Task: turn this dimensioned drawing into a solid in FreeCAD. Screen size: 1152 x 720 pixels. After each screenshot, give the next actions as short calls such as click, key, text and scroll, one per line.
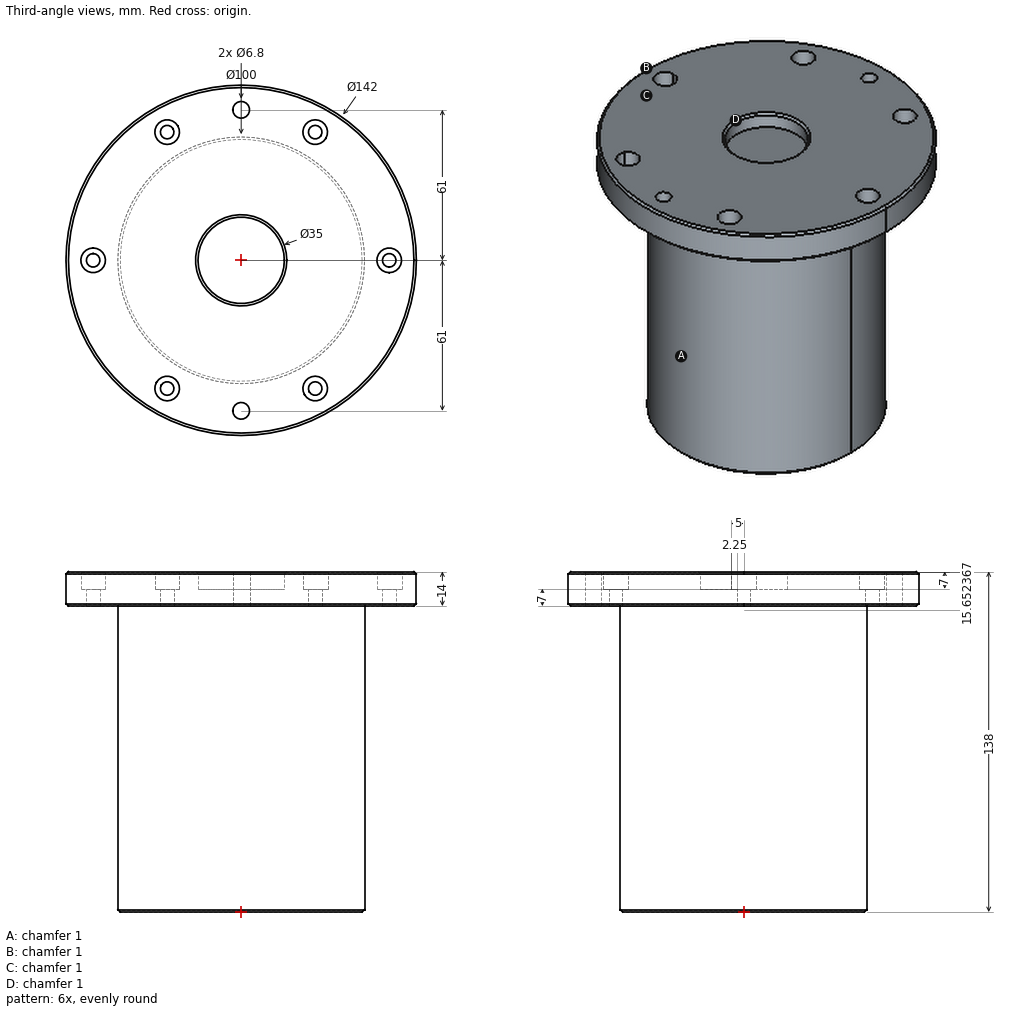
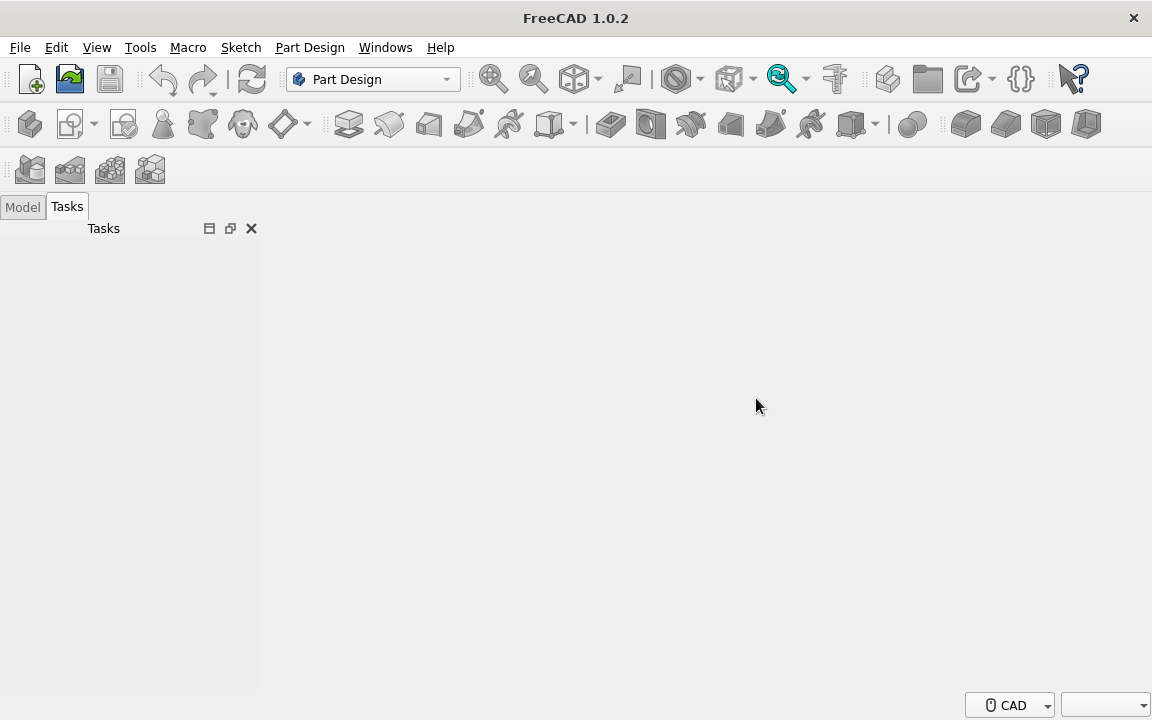
click(30, 80)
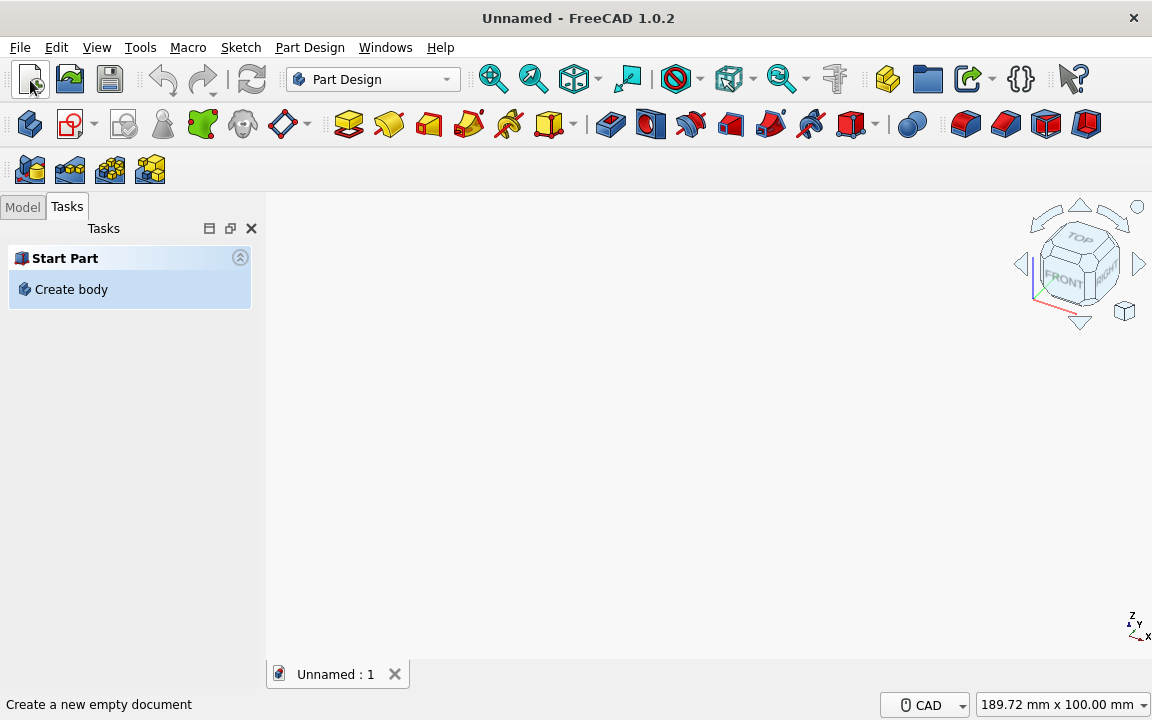
click(70, 124)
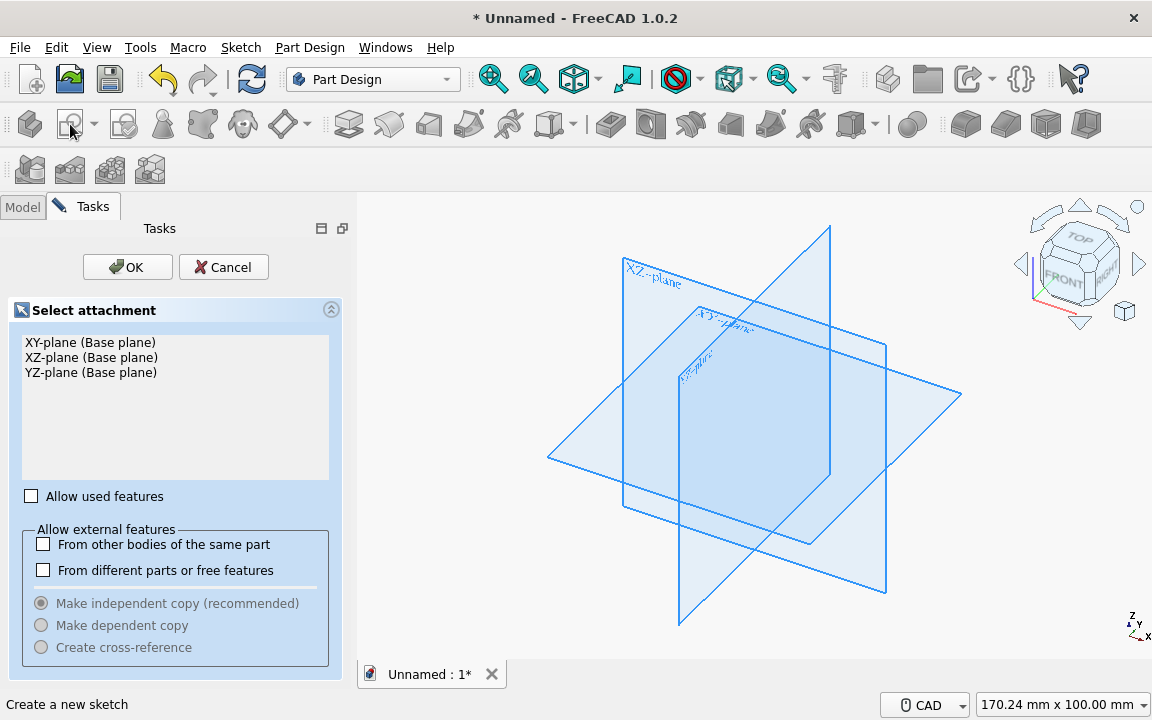
click(82, 342)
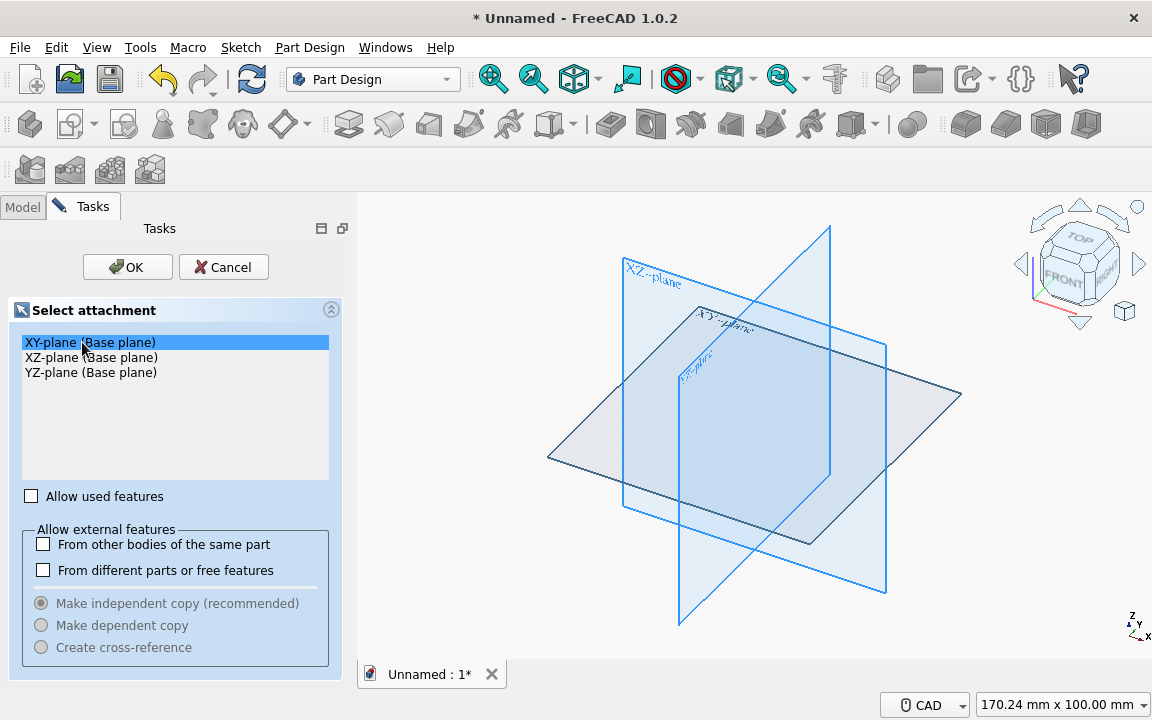
click(128, 267)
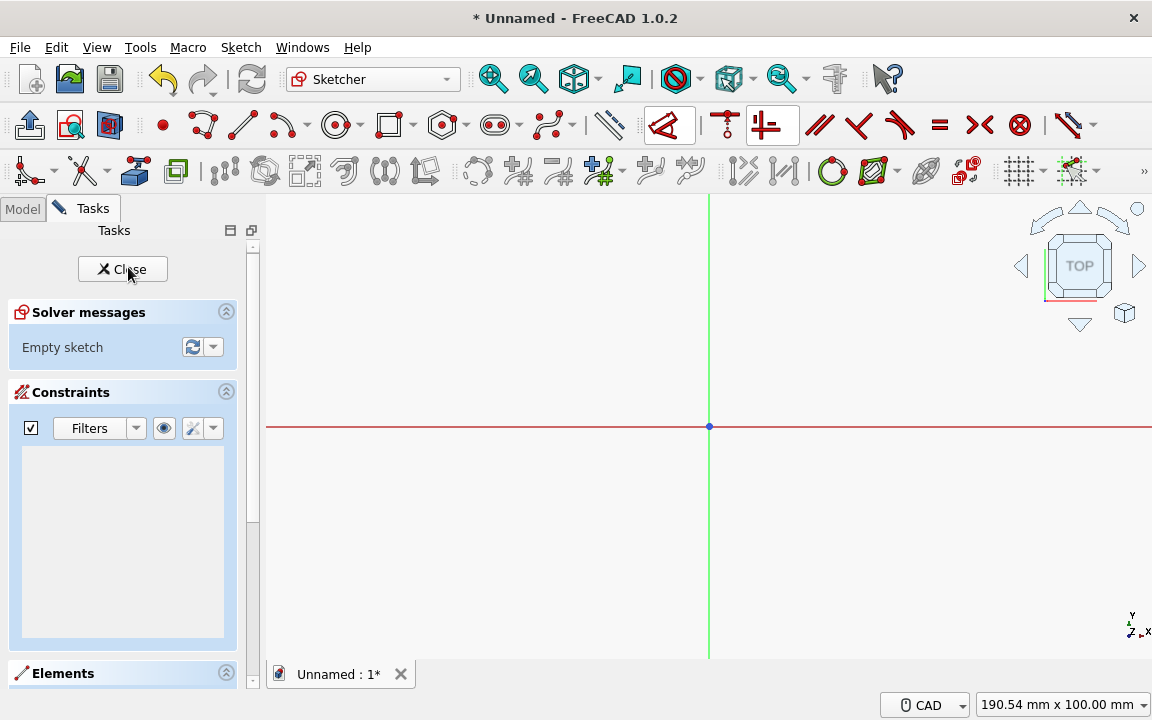
scroll(501, 427, down, 2)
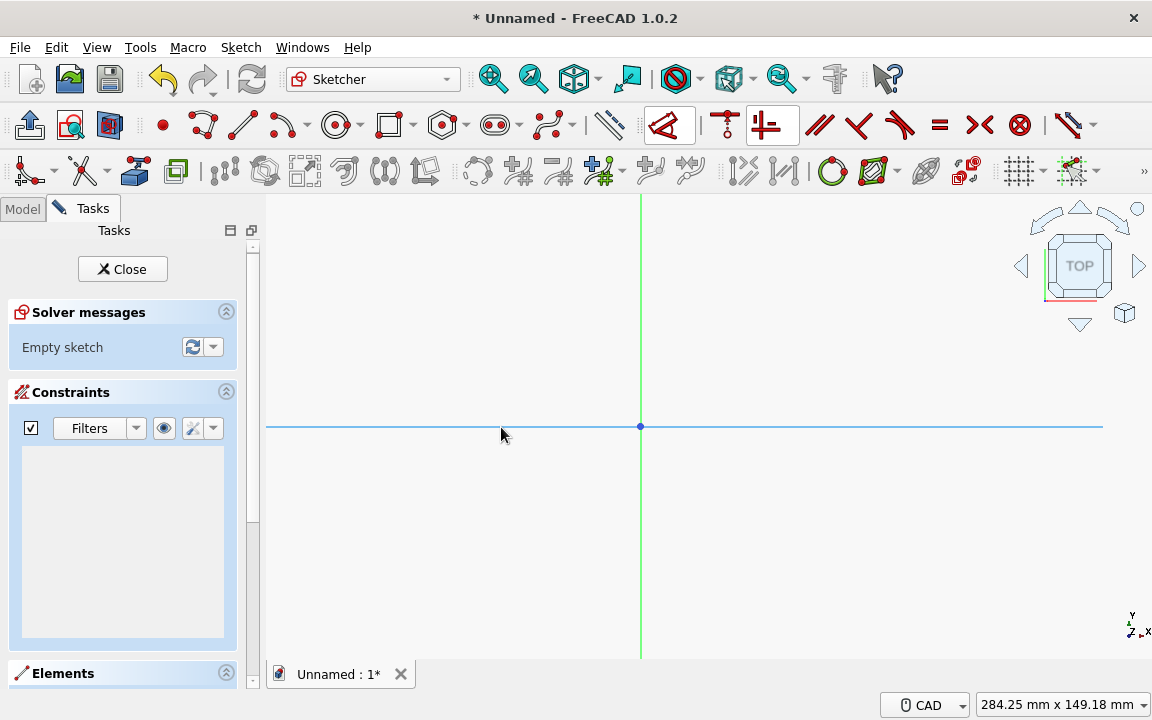
key(g)
key(c)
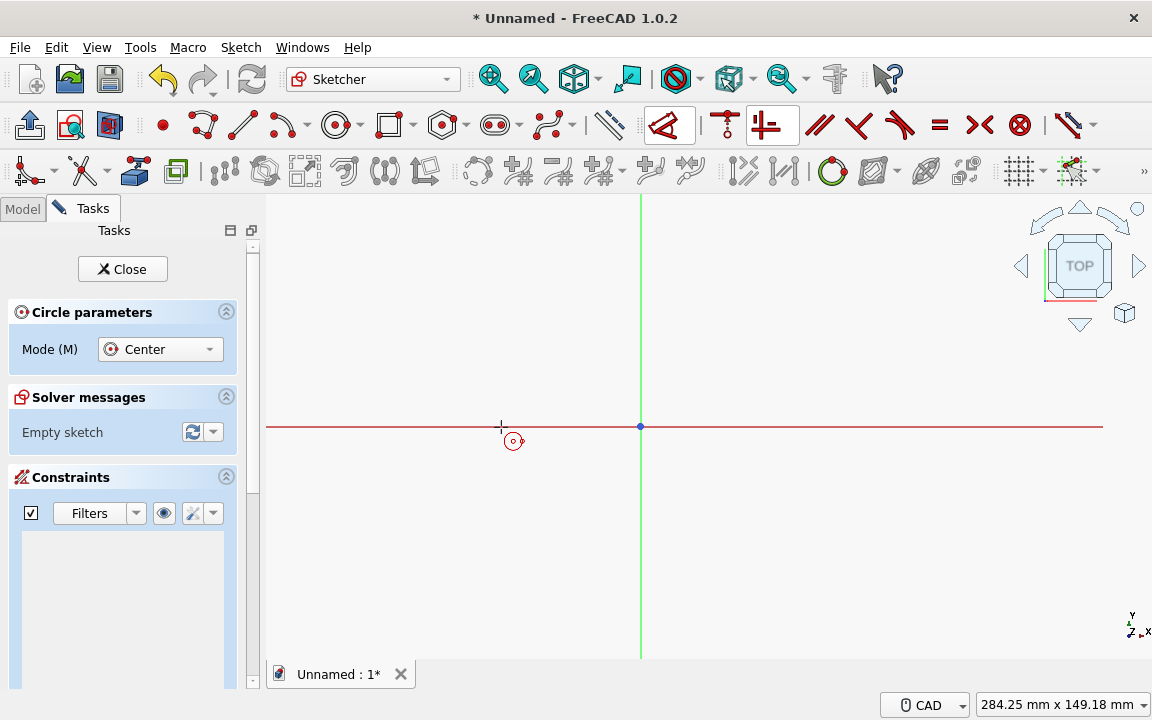
click(641, 427)
click(751, 317)
key(Escape)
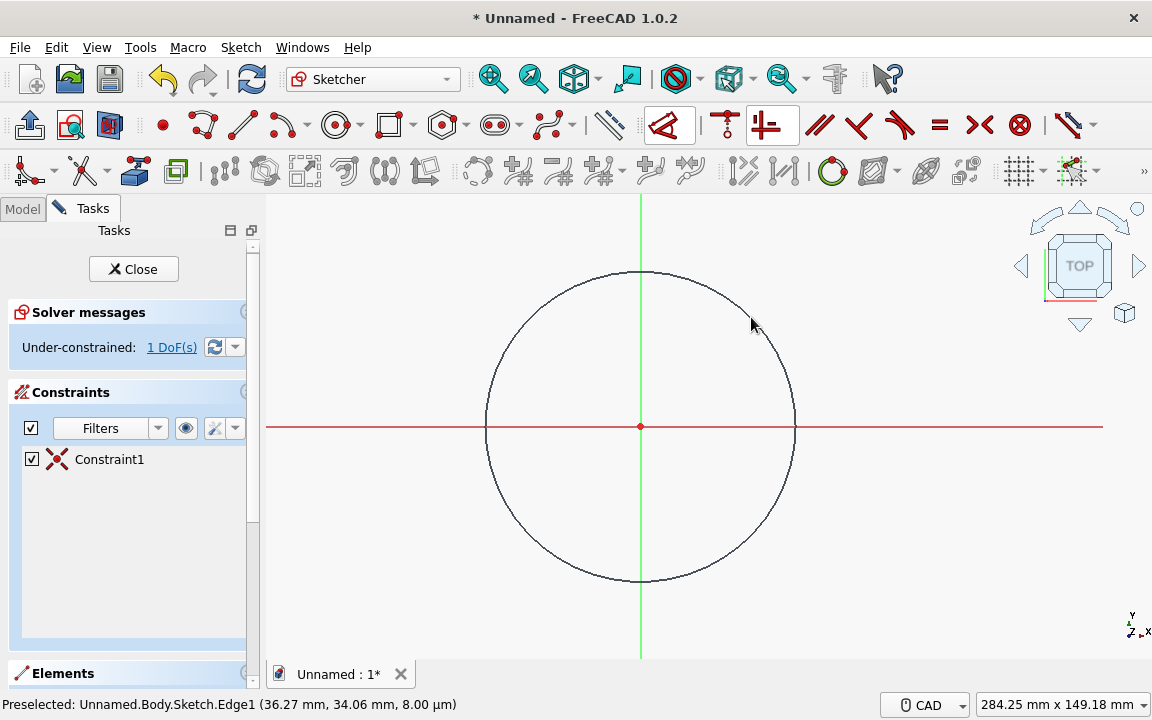
click(750, 317)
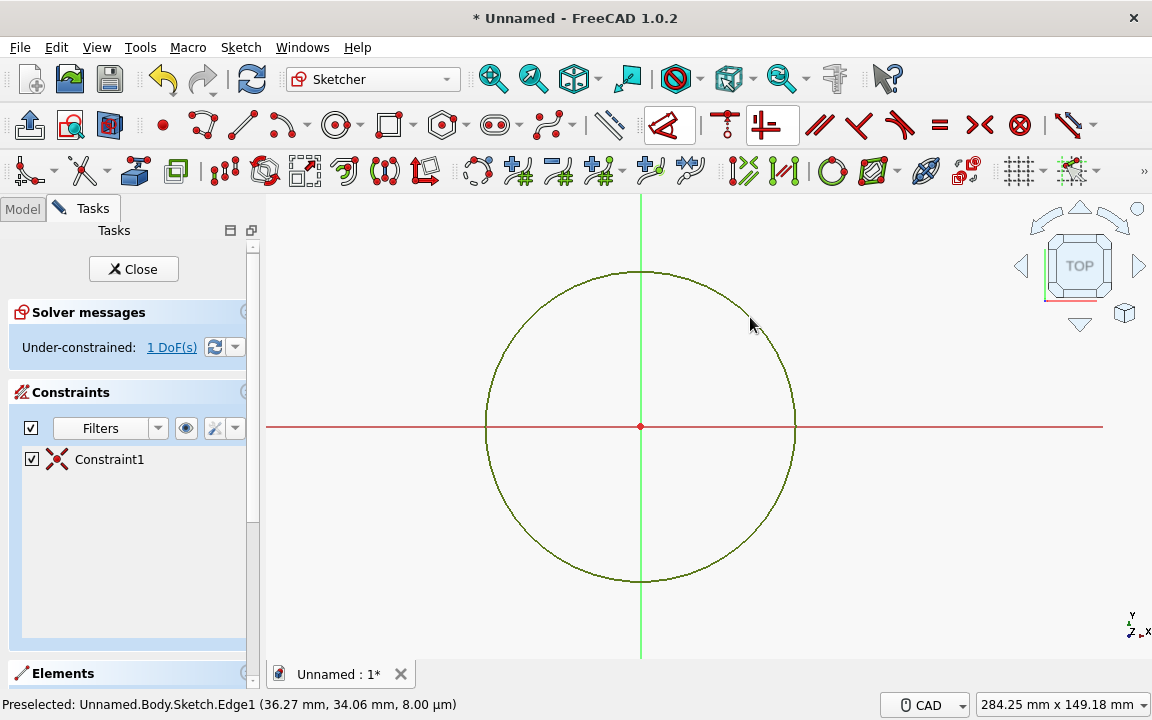
key(k)
key(o)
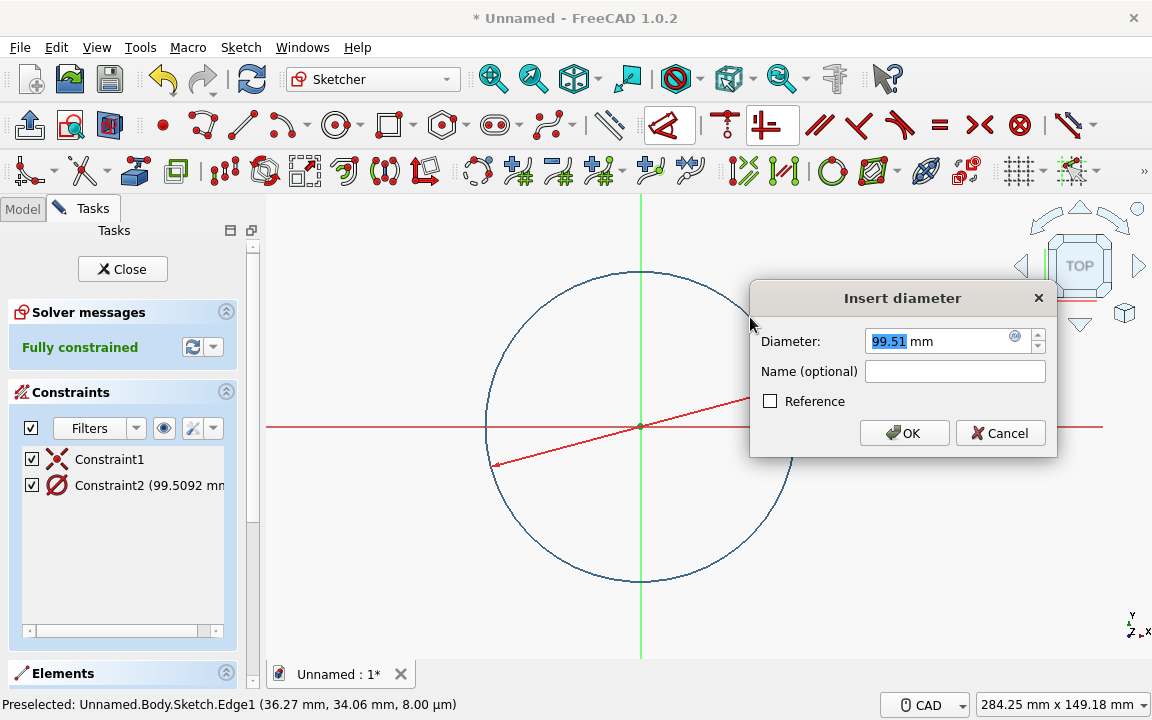
text(100)
key(Return)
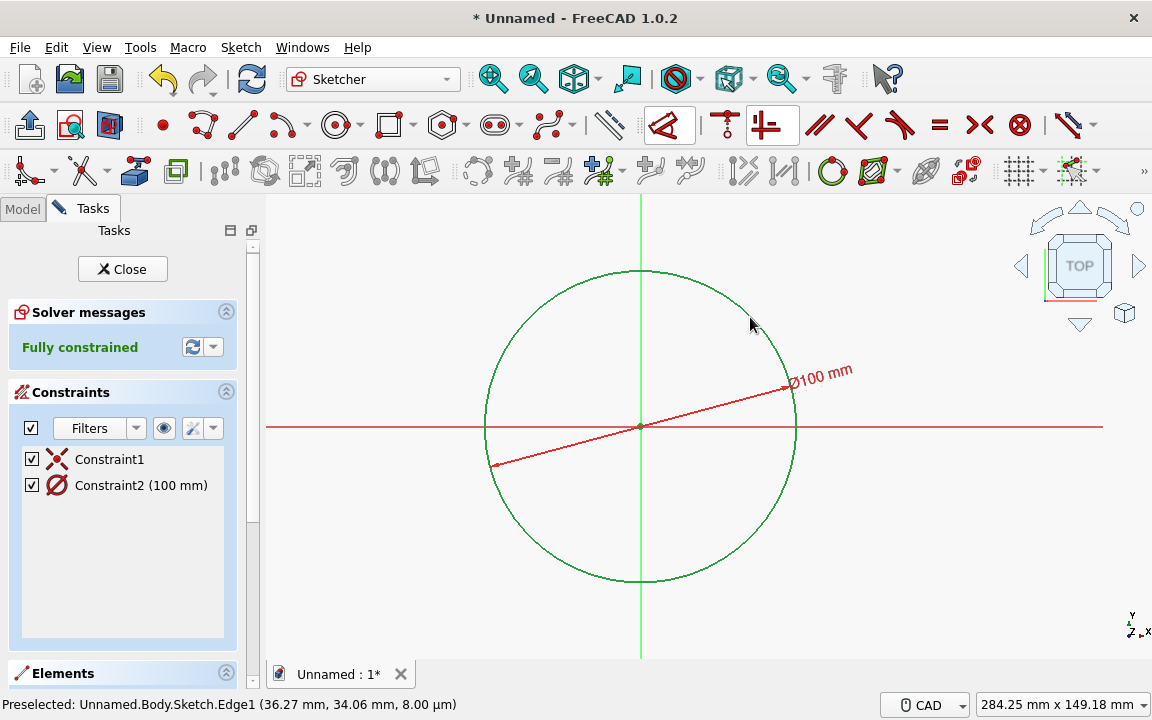
click(123, 269)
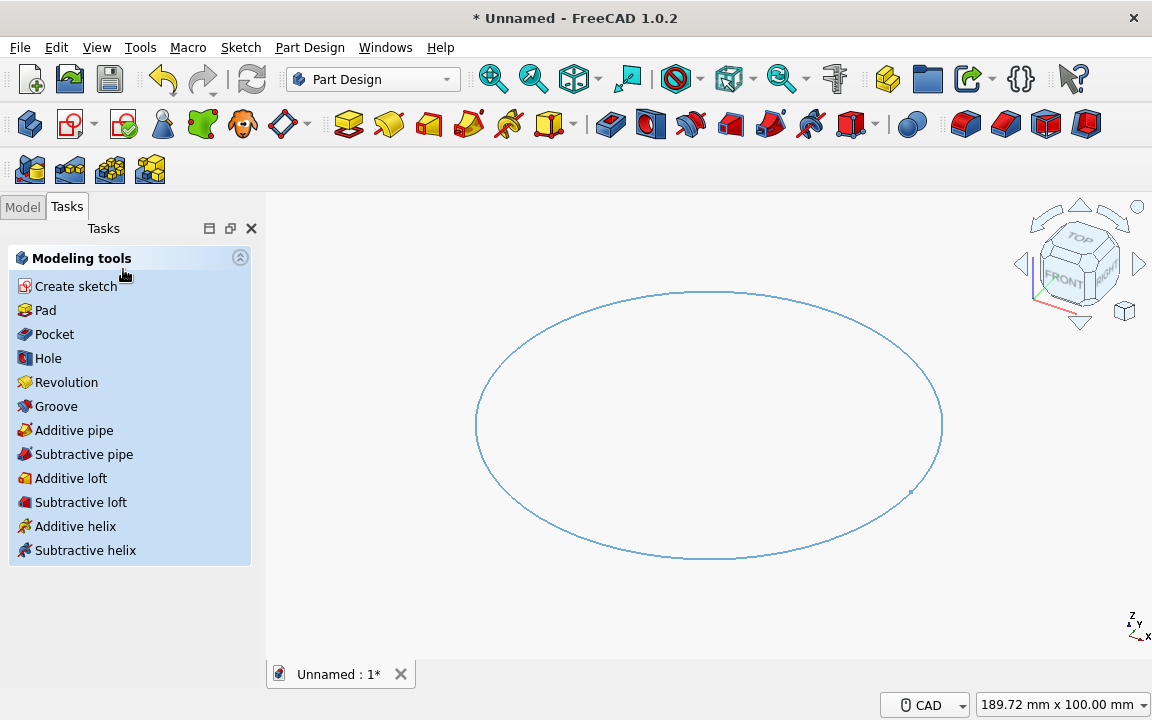
click(350, 124)